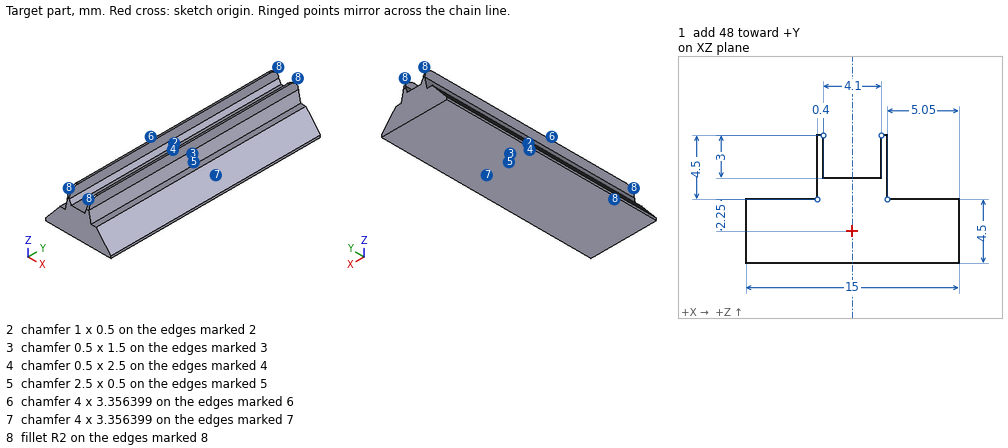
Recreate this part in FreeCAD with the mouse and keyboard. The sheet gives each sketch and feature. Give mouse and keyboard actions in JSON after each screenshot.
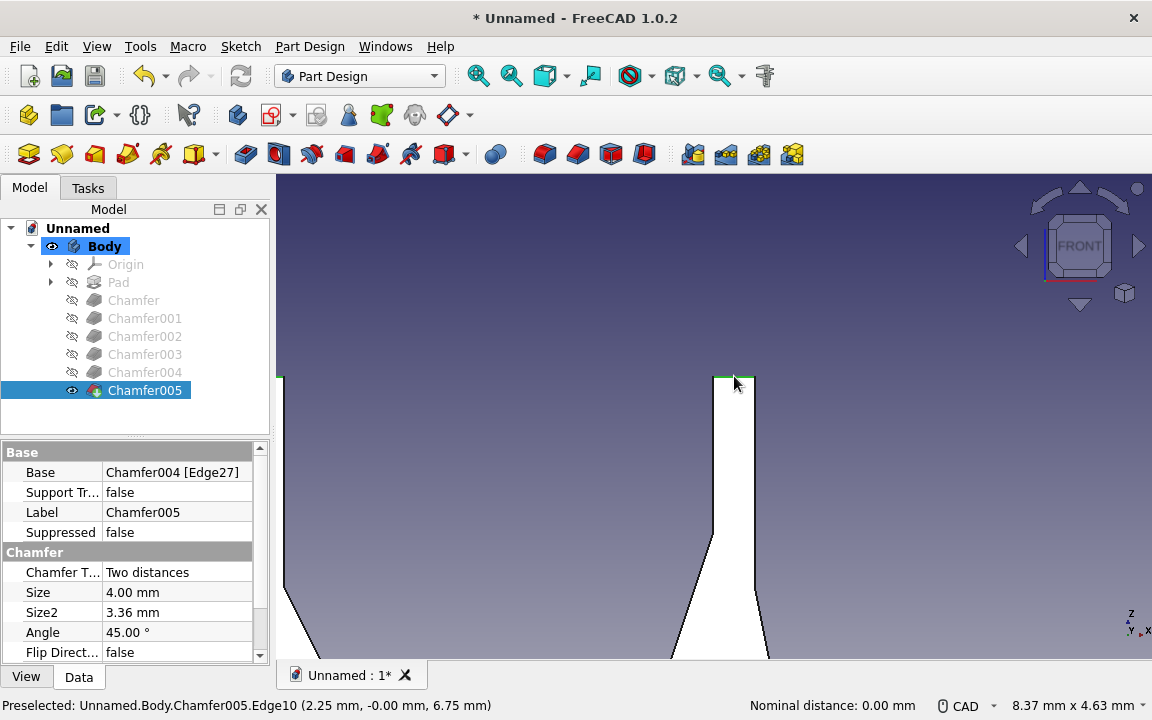
{"action": "left_click", "coordinate": [479, 76]}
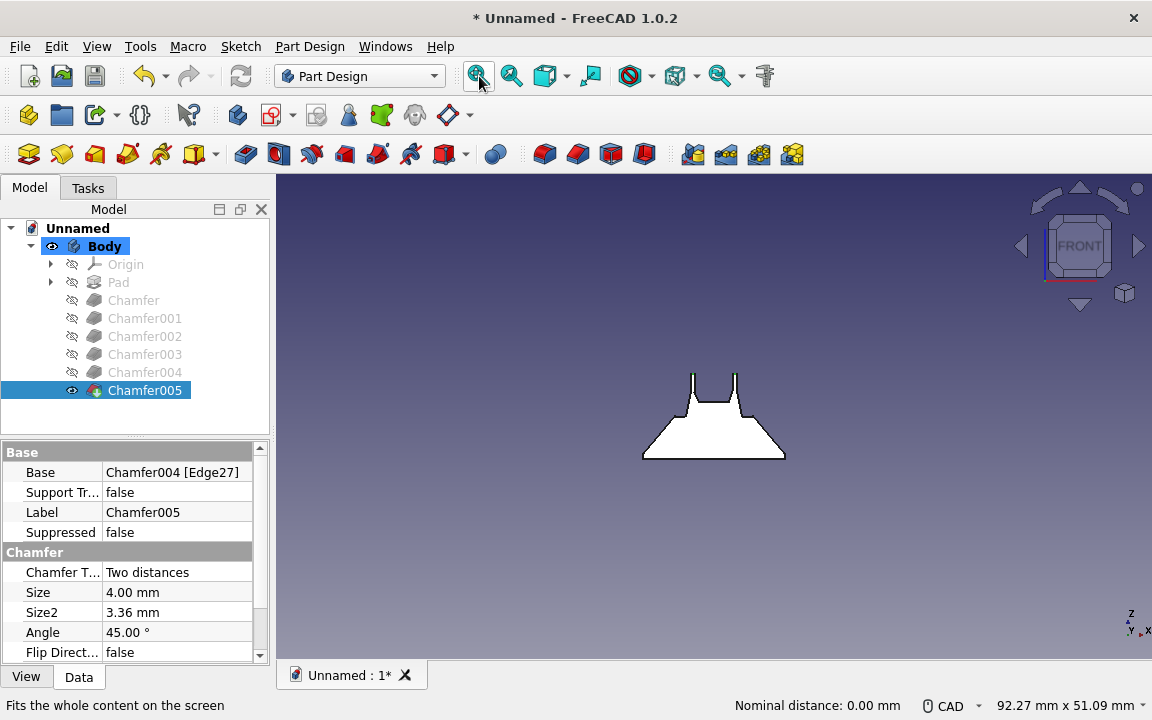
{"action": "key", "text": "3"}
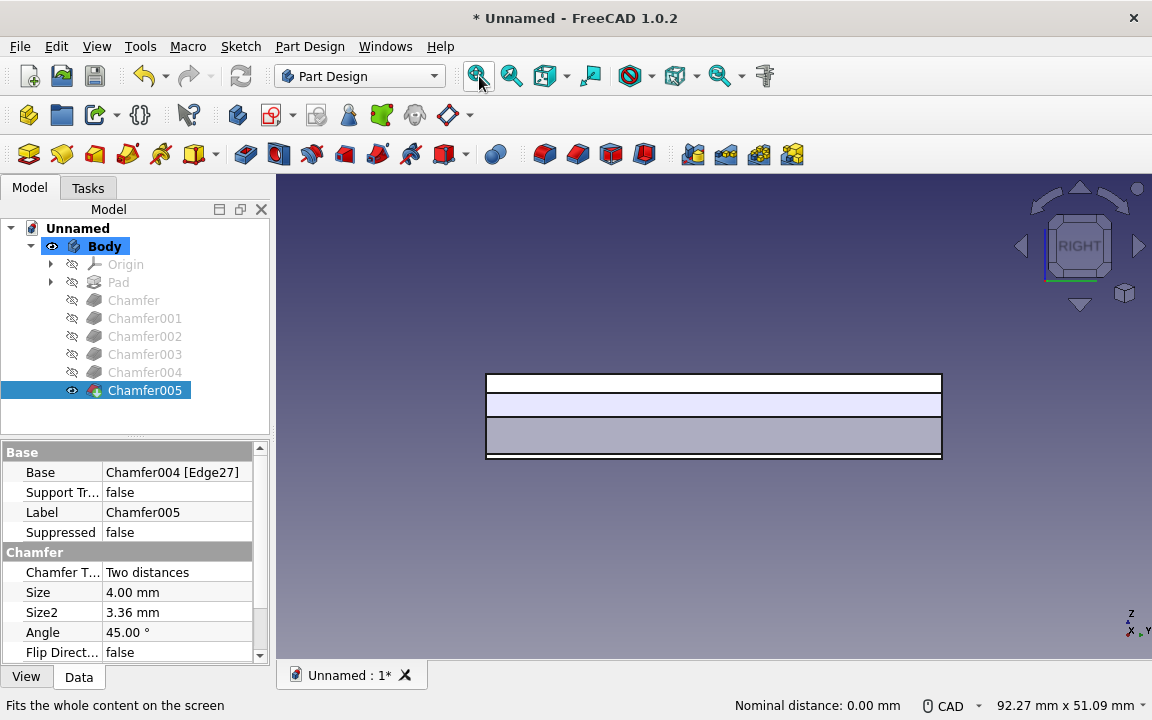
{"action": "scroll", "coordinate": [942, 373], "scroll_direction": "up", "scroll_amount": 12}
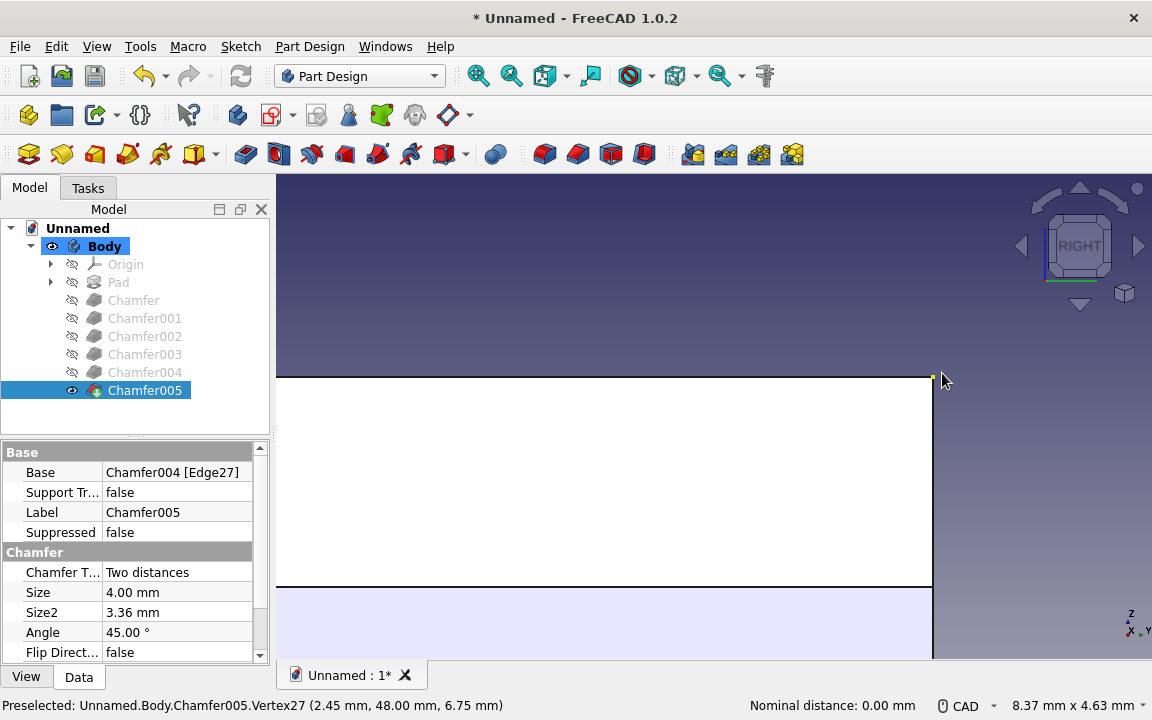
{"action": "left_click", "coordinate": [479, 76]}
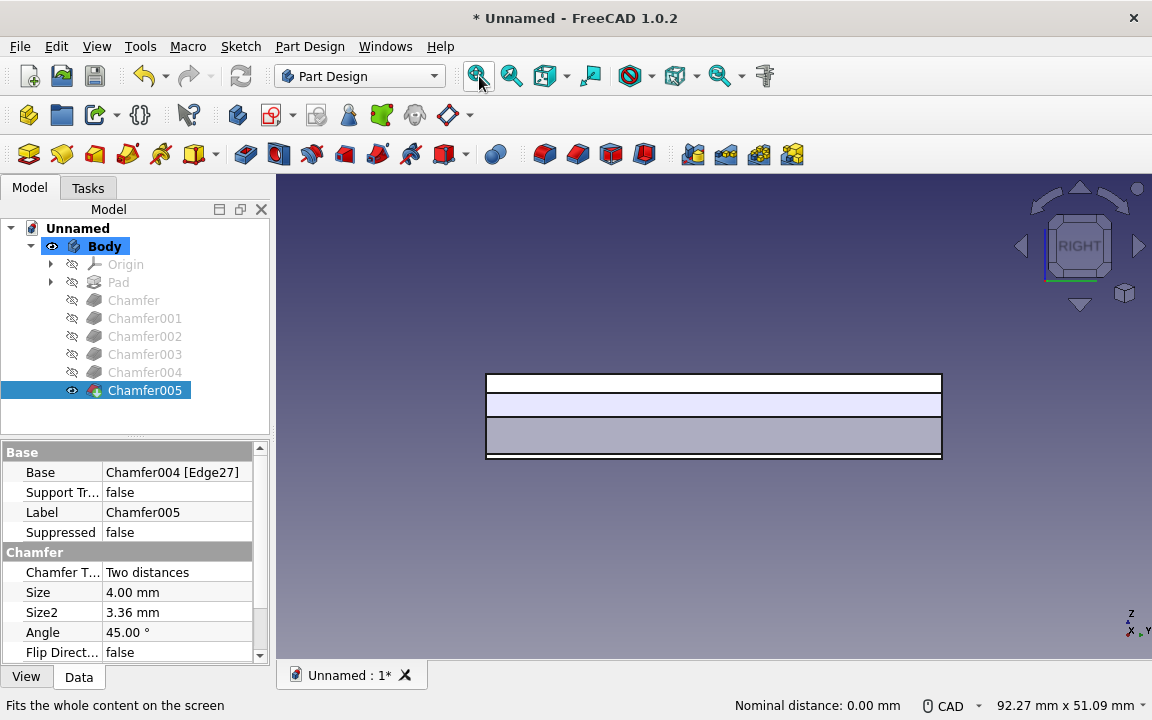
{"action": "key", "text": "5"}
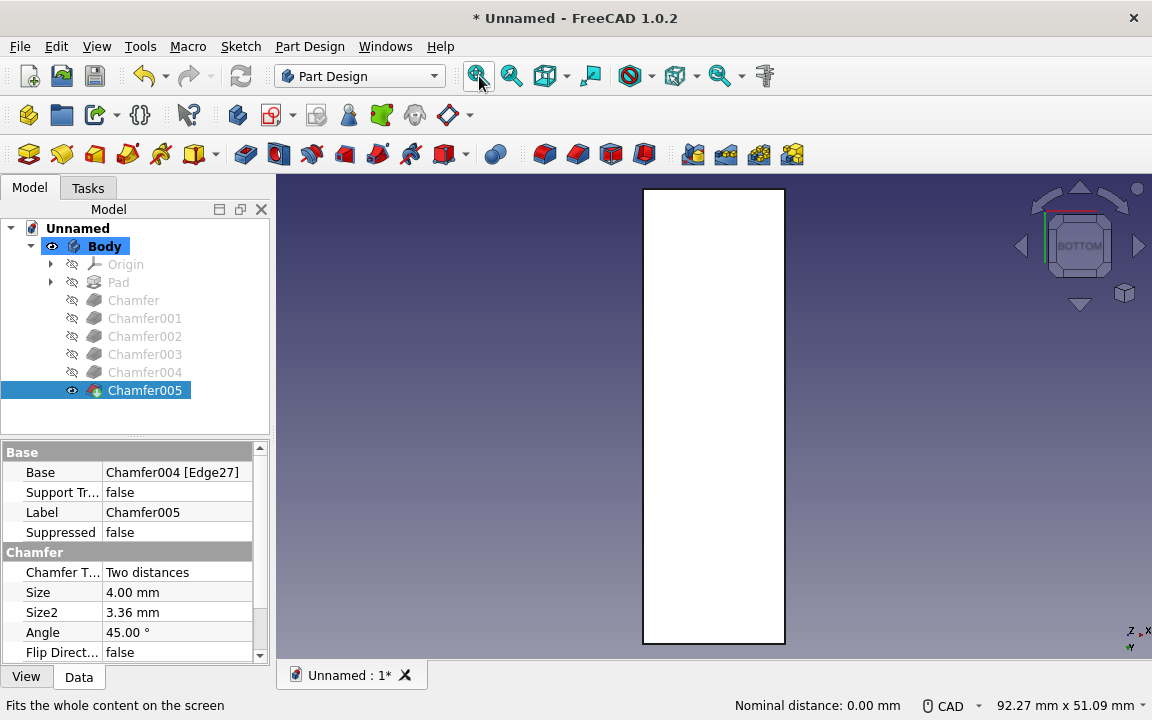
{"action": "key", "text": "4"}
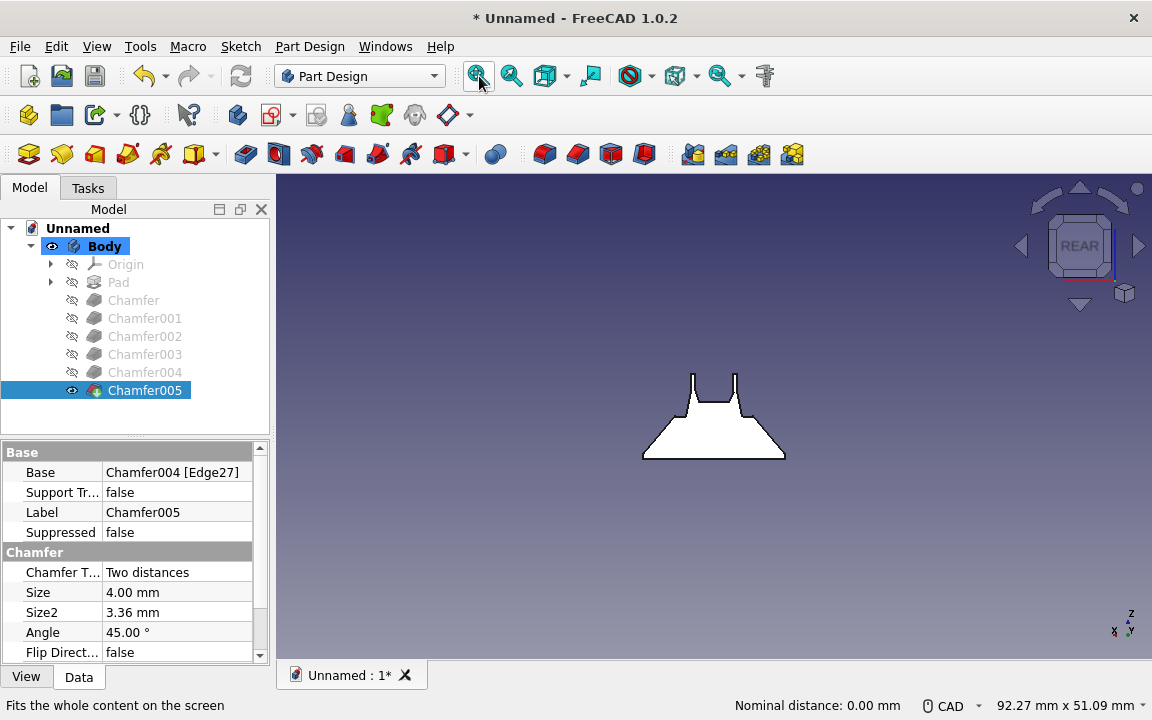
{"action": "left_click", "coordinate": [479, 76]}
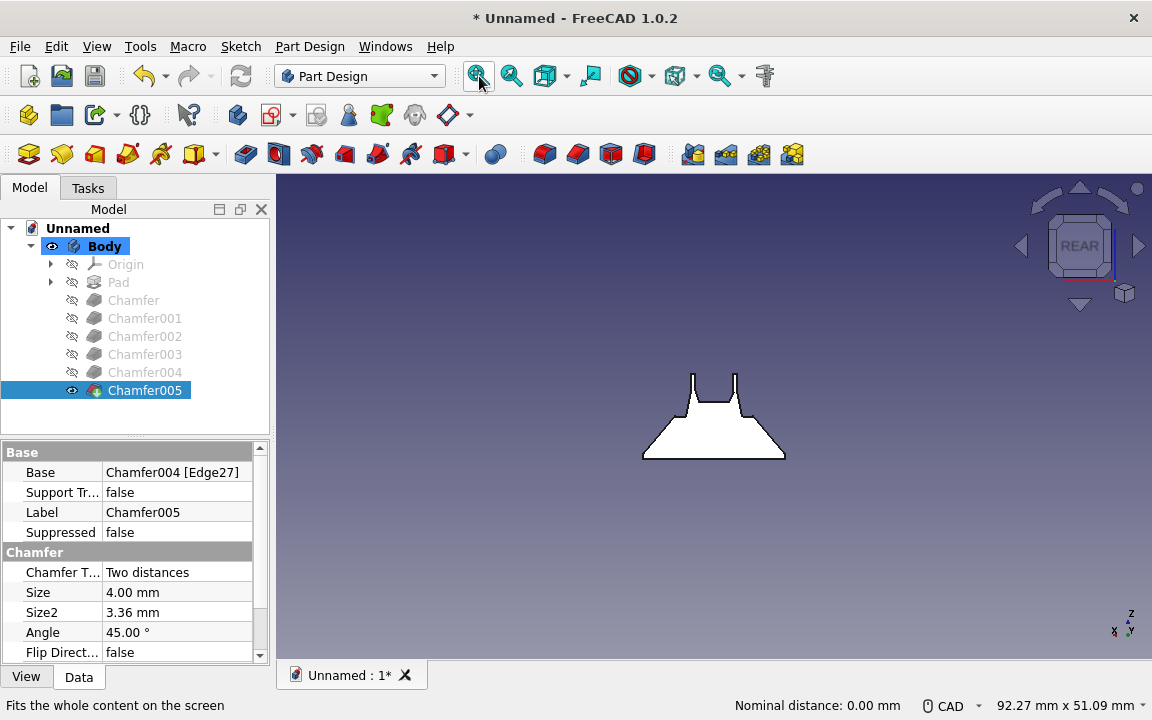
{"action": "scroll", "coordinate": [735, 373], "scroll_direction": "up", "scroll_amount": 12}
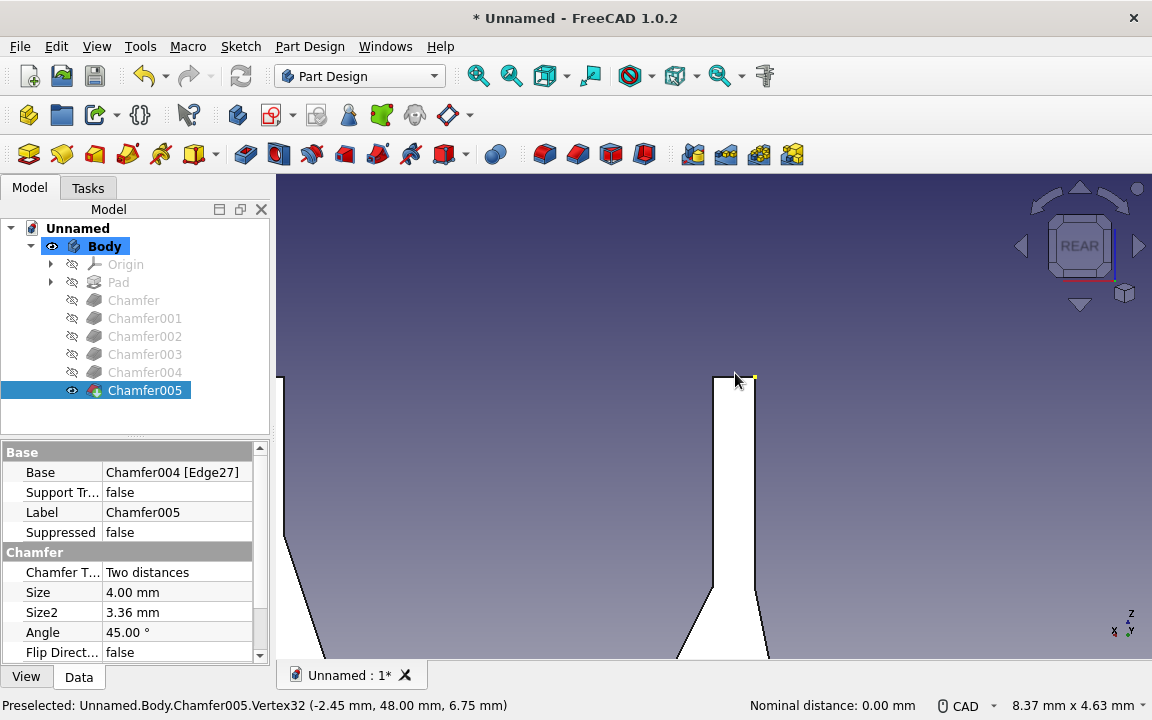
{"action": "key", "text": "v f"}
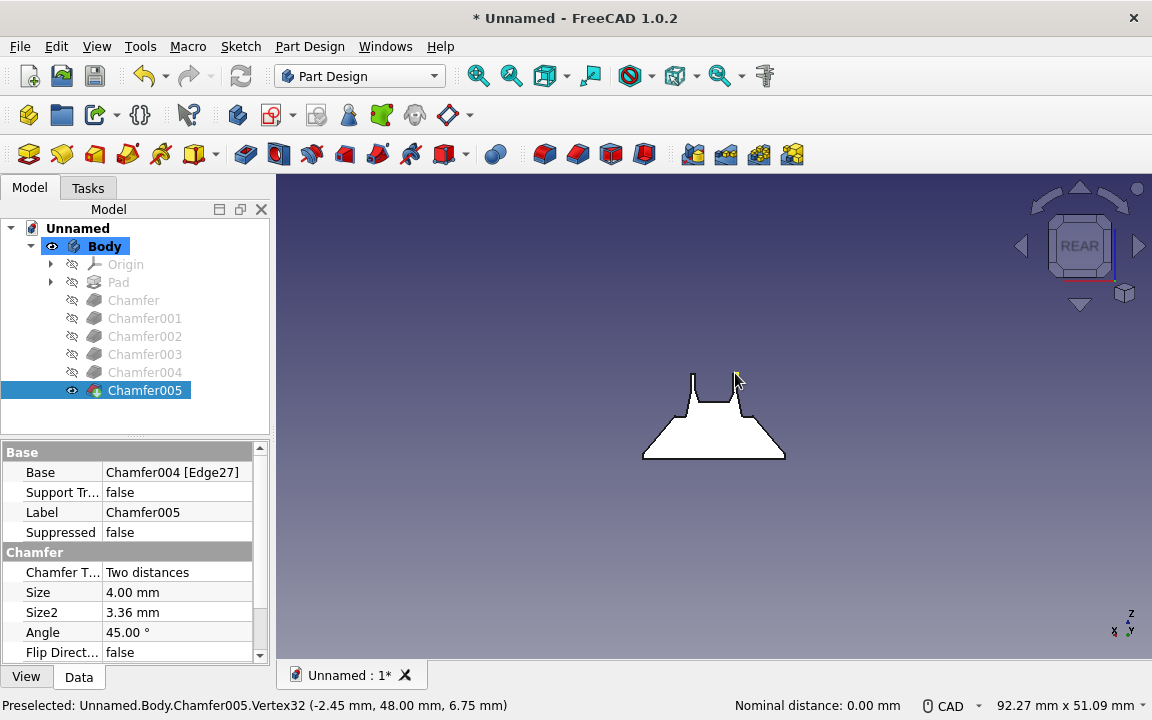
{"action": "key", "text": "6"}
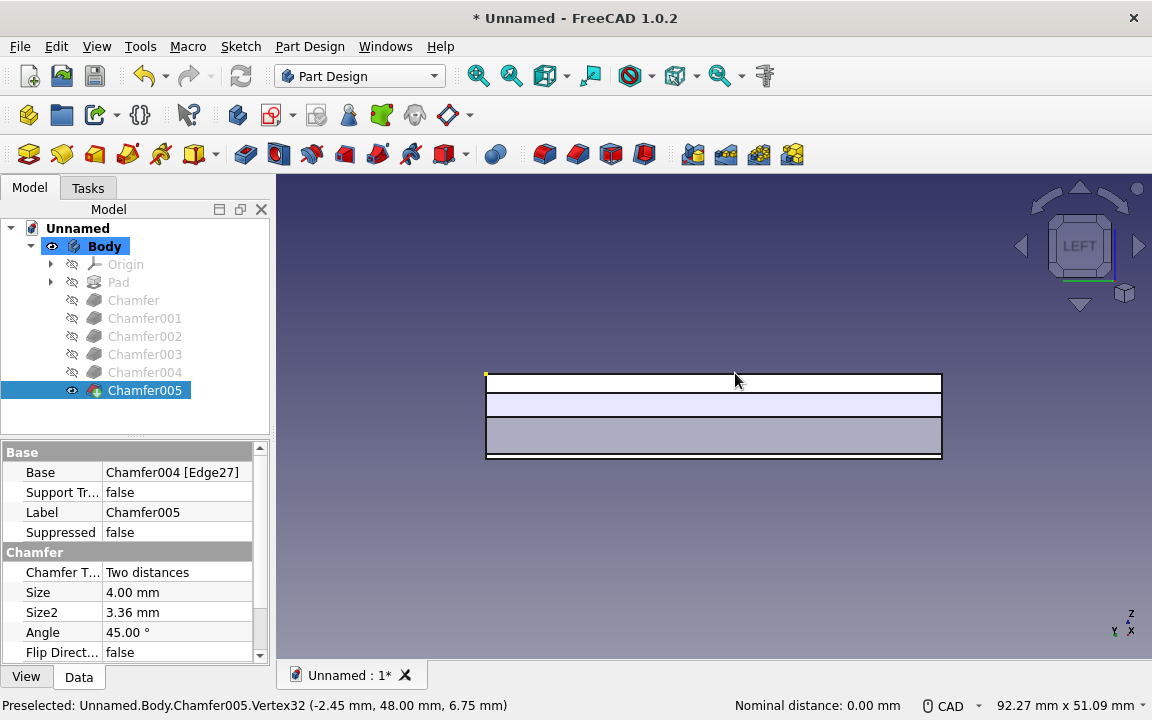
{"action": "scroll", "coordinate": [486, 373], "scroll_direction": "up", "scroll_amount": 12}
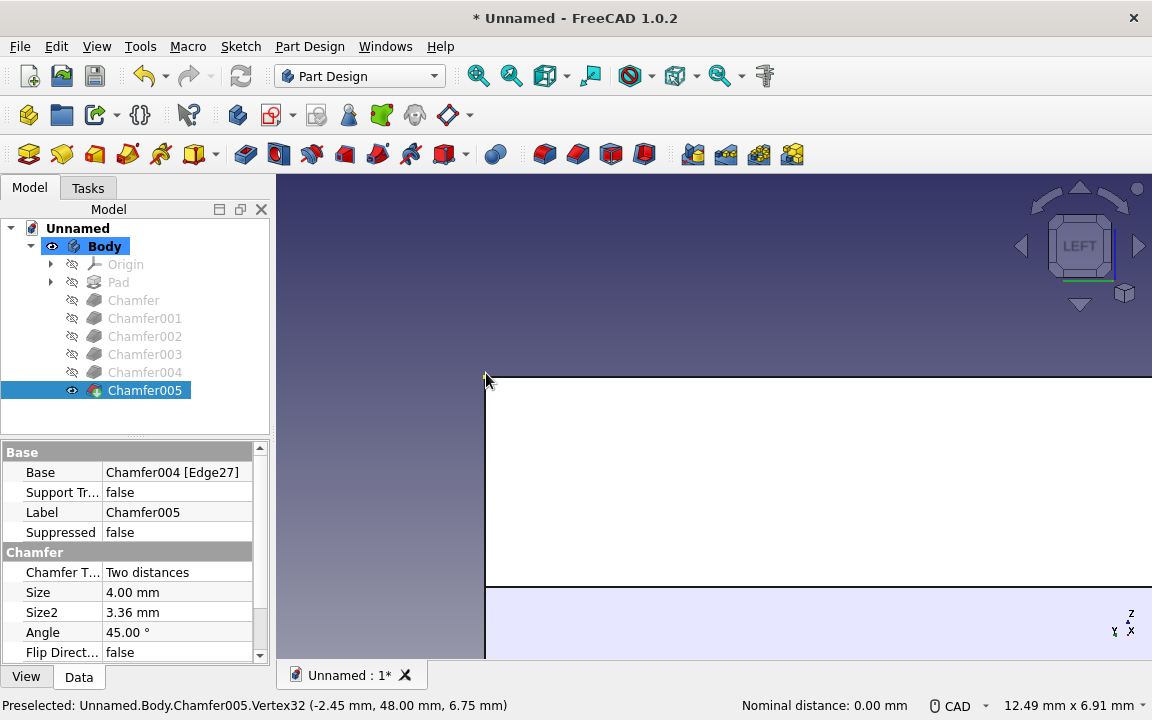
{"action": "left_click", "coordinate": [479, 76]}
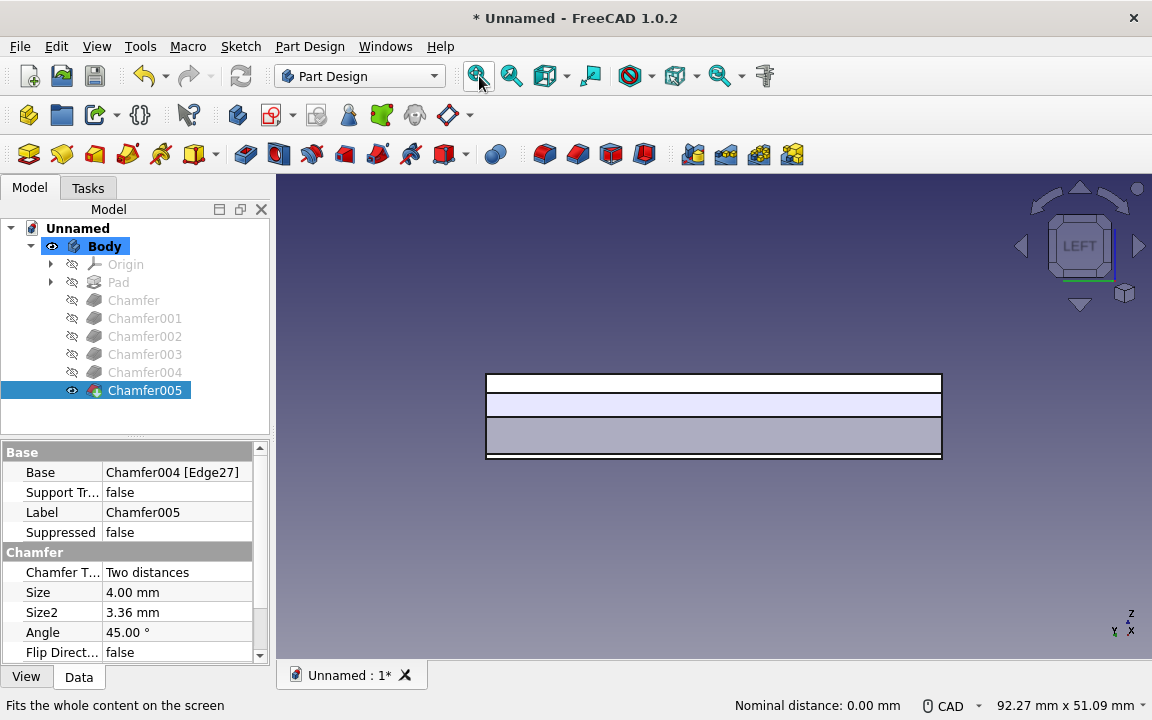
{"action": "key", "text": "v 3"}